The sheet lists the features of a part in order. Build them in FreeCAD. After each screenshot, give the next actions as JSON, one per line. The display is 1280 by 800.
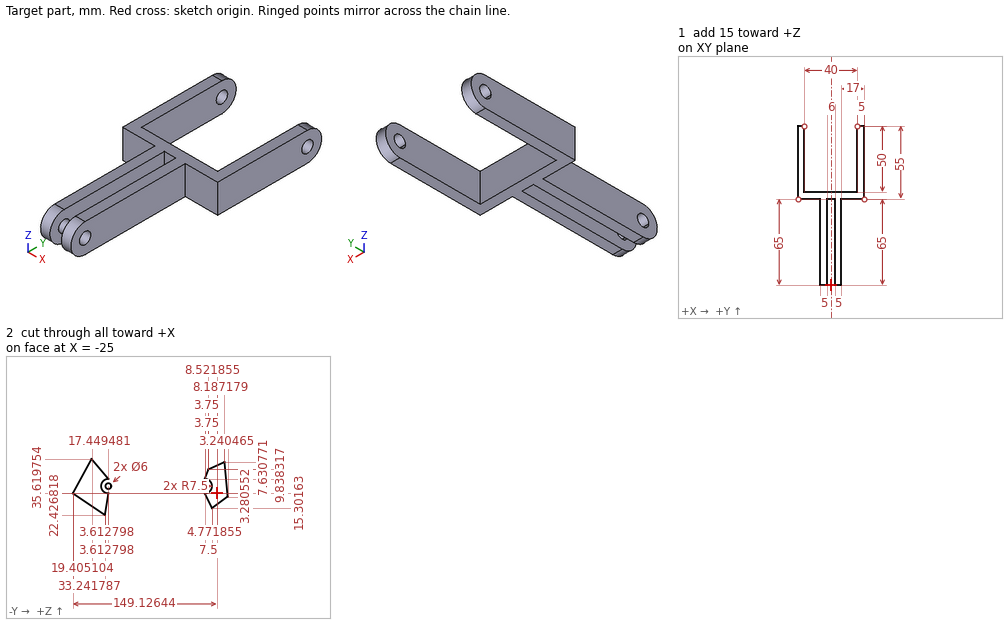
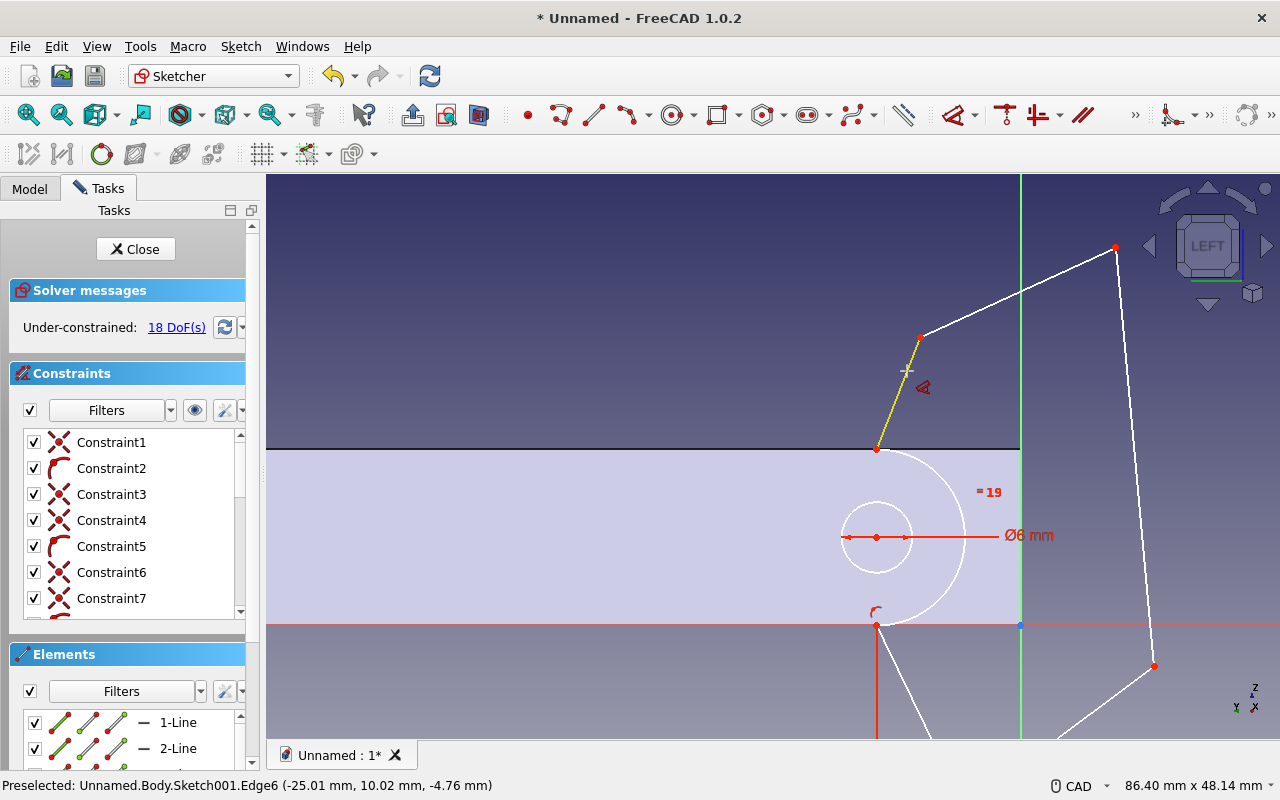
{"action": "left_click", "coordinate": [907, 371]}
{"action": "left_click", "coordinate": [898, 304]}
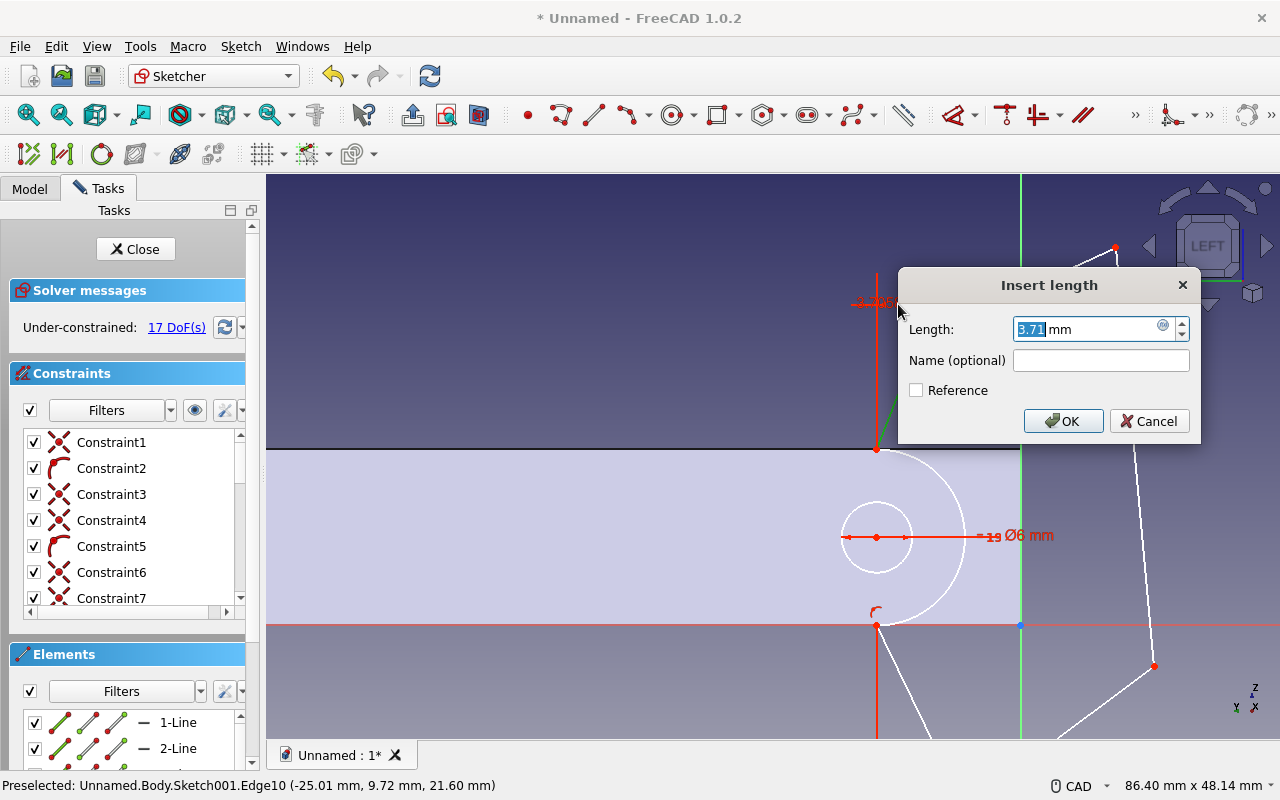
{"action": "type", "text": "3.75"}
{"action": "key", "text": "Return"}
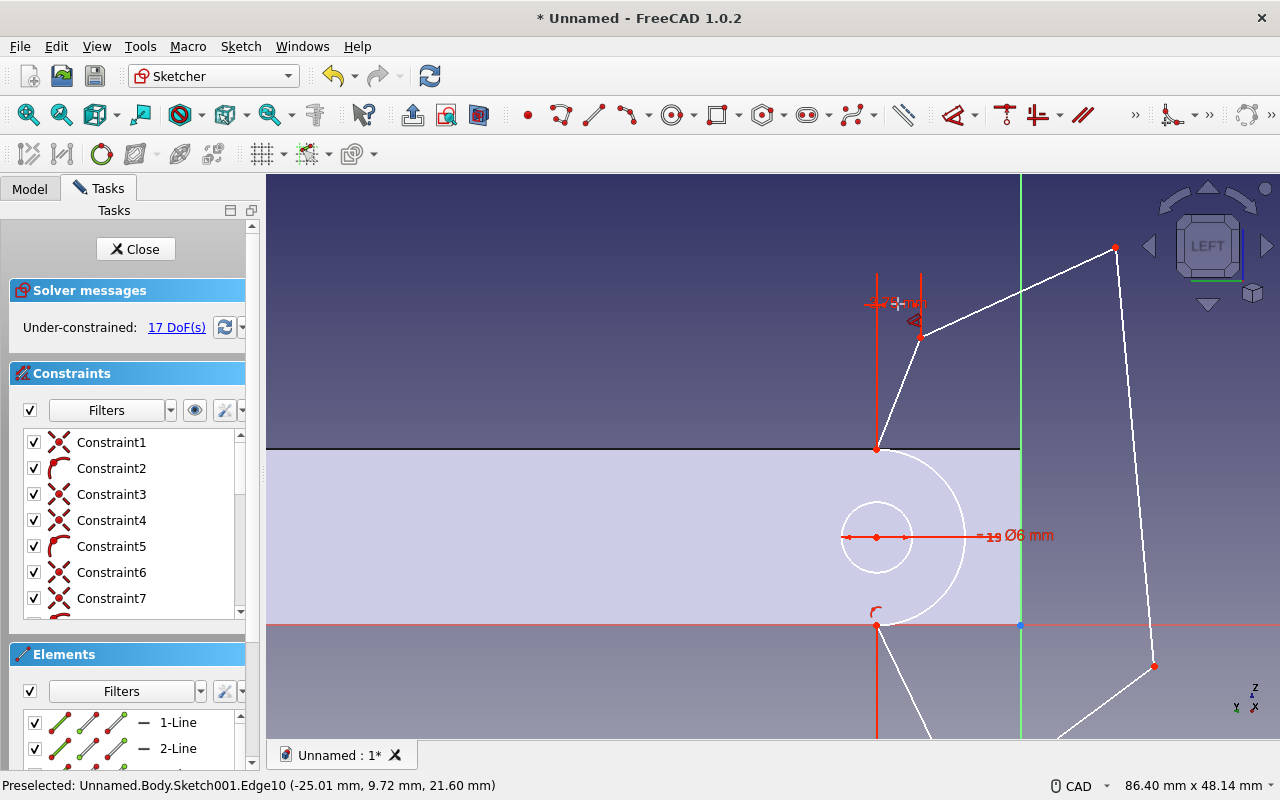
{"action": "left_click", "coordinate": [921, 338]}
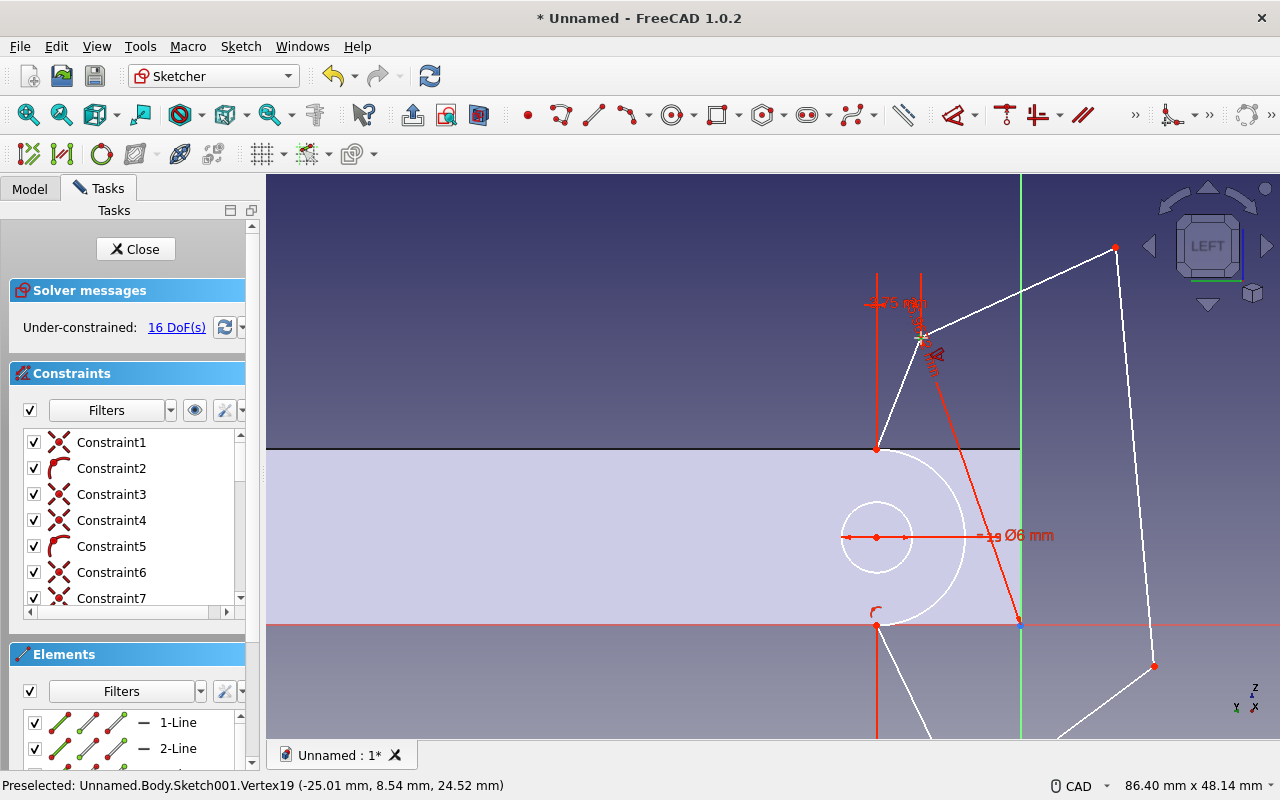
{"action": "left_click", "coordinate": [877, 537]}
{"action": "left_click", "coordinate": [914, 571]}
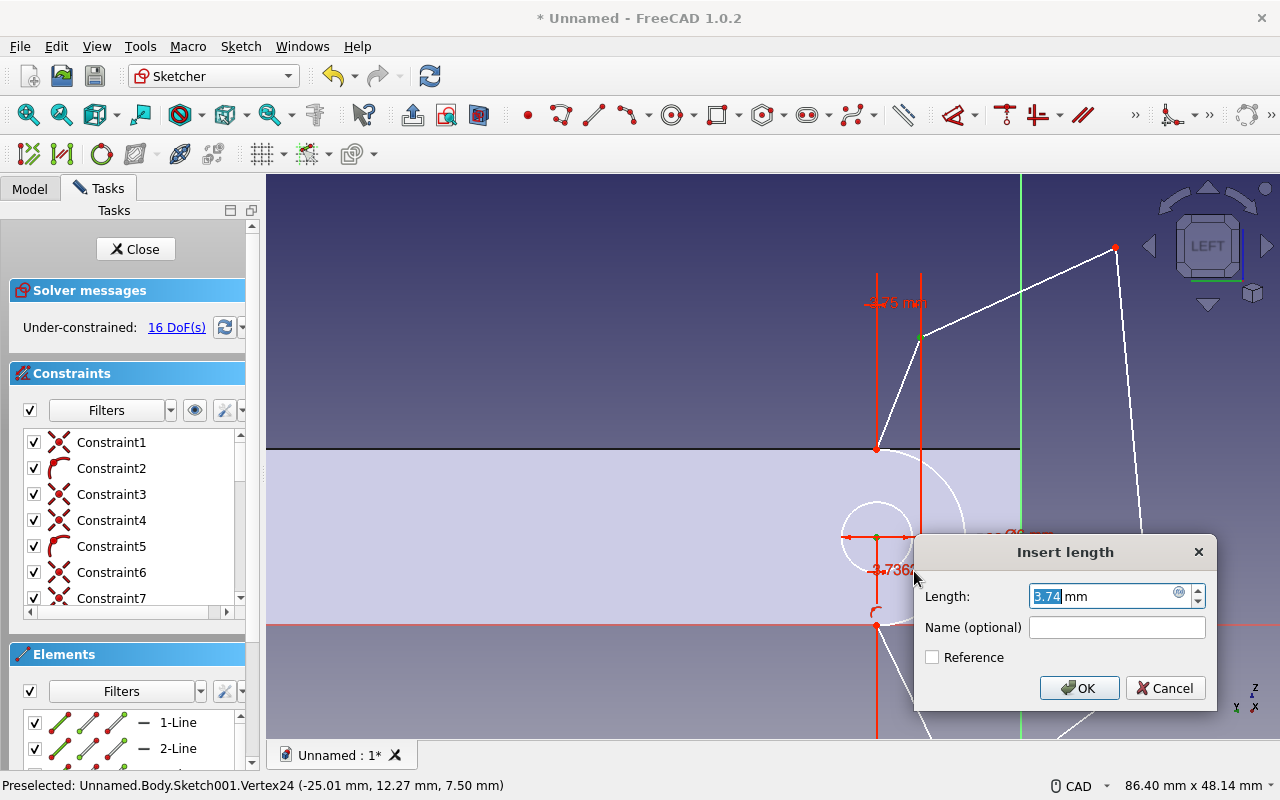
{"action": "type", "text": "3.75"}
{"action": "key", "text": "Return"}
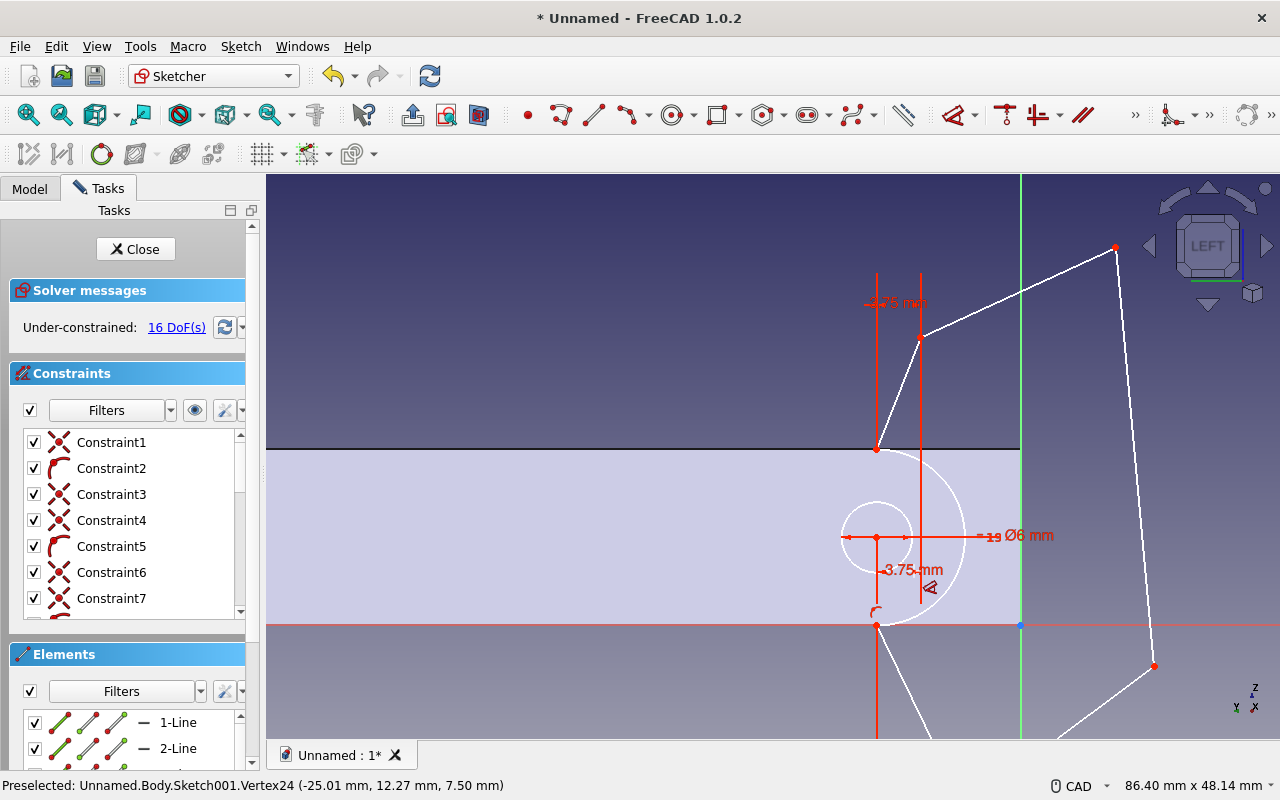
{"action": "scroll", "coordinate": [916, 417], "scroll_direction": "down", "scroll_amount": 6}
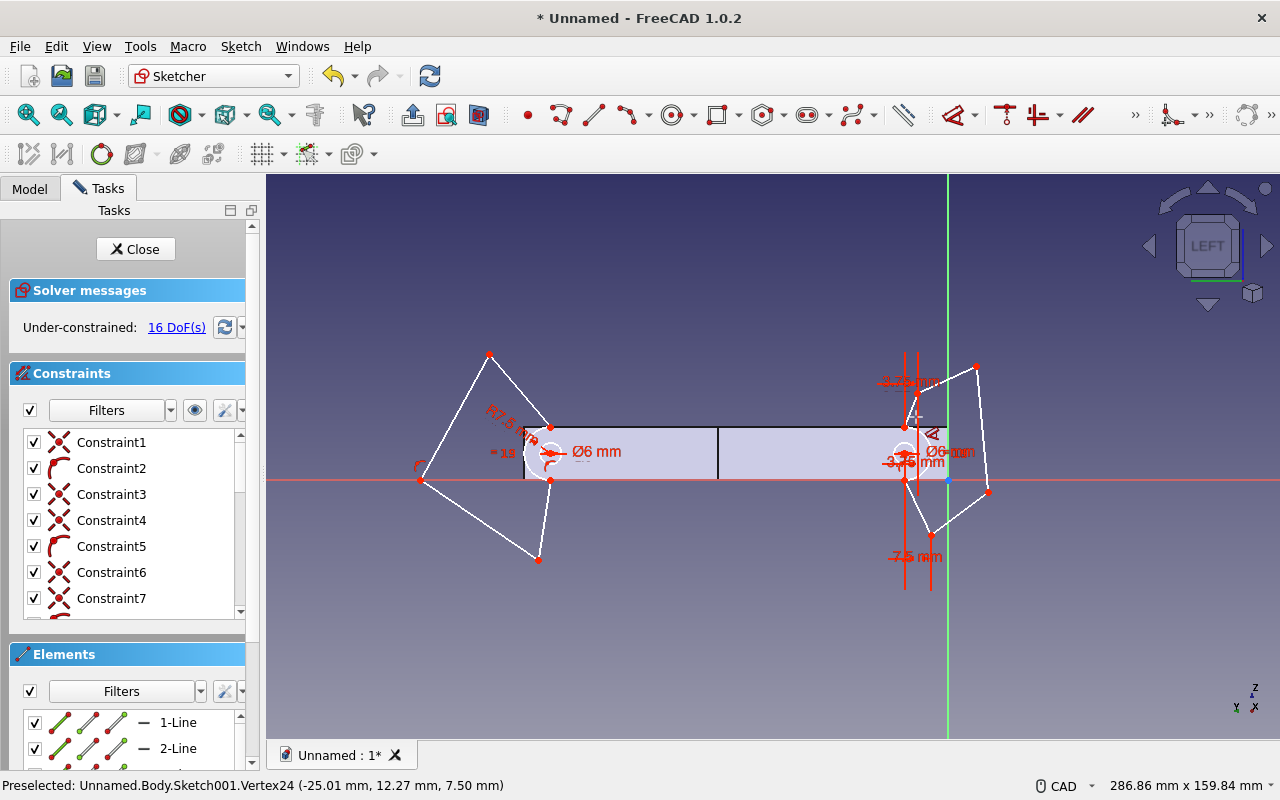
{"action": "scroll", "coordinate": [931, 535], "scroll_direction": "up", "scroll_amount": 5}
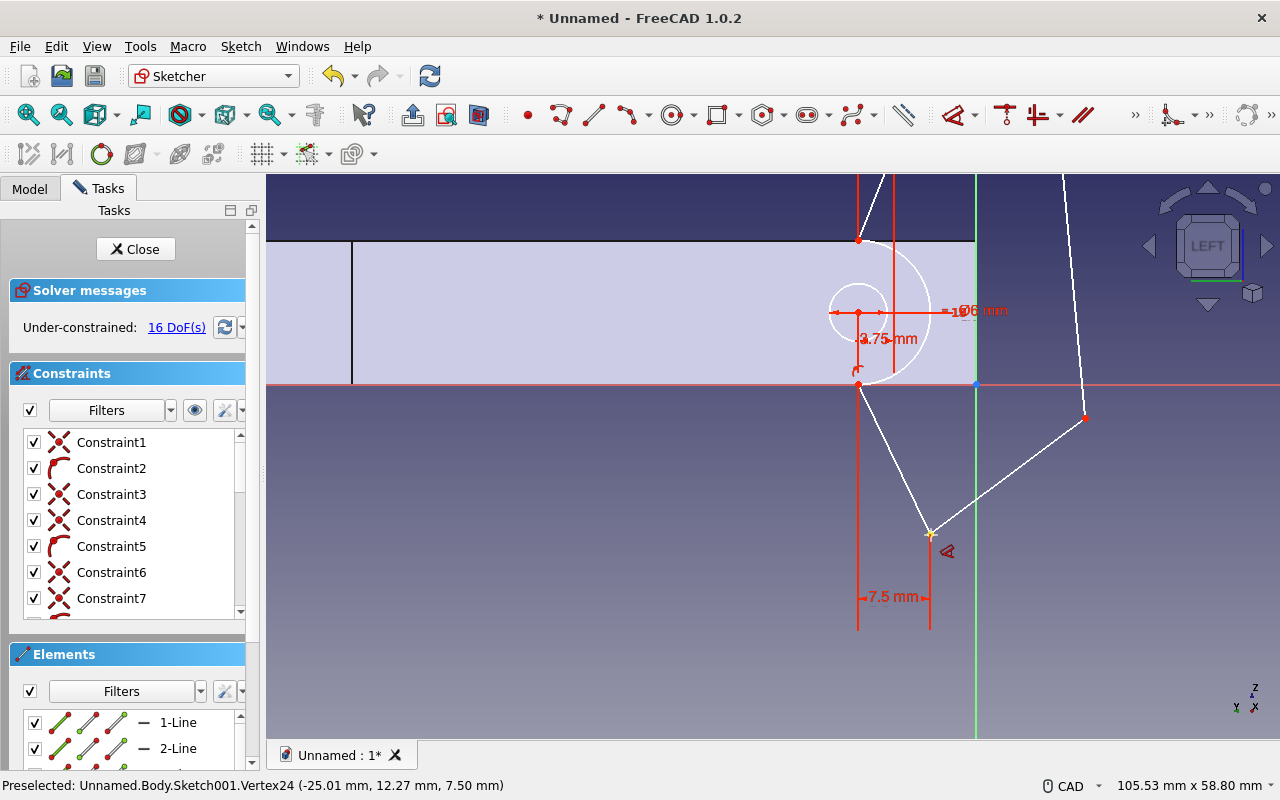
{"action": "left_click", "coordinate": [930, 534]}
{"action": "left_click", "coordinate": [953, 568]}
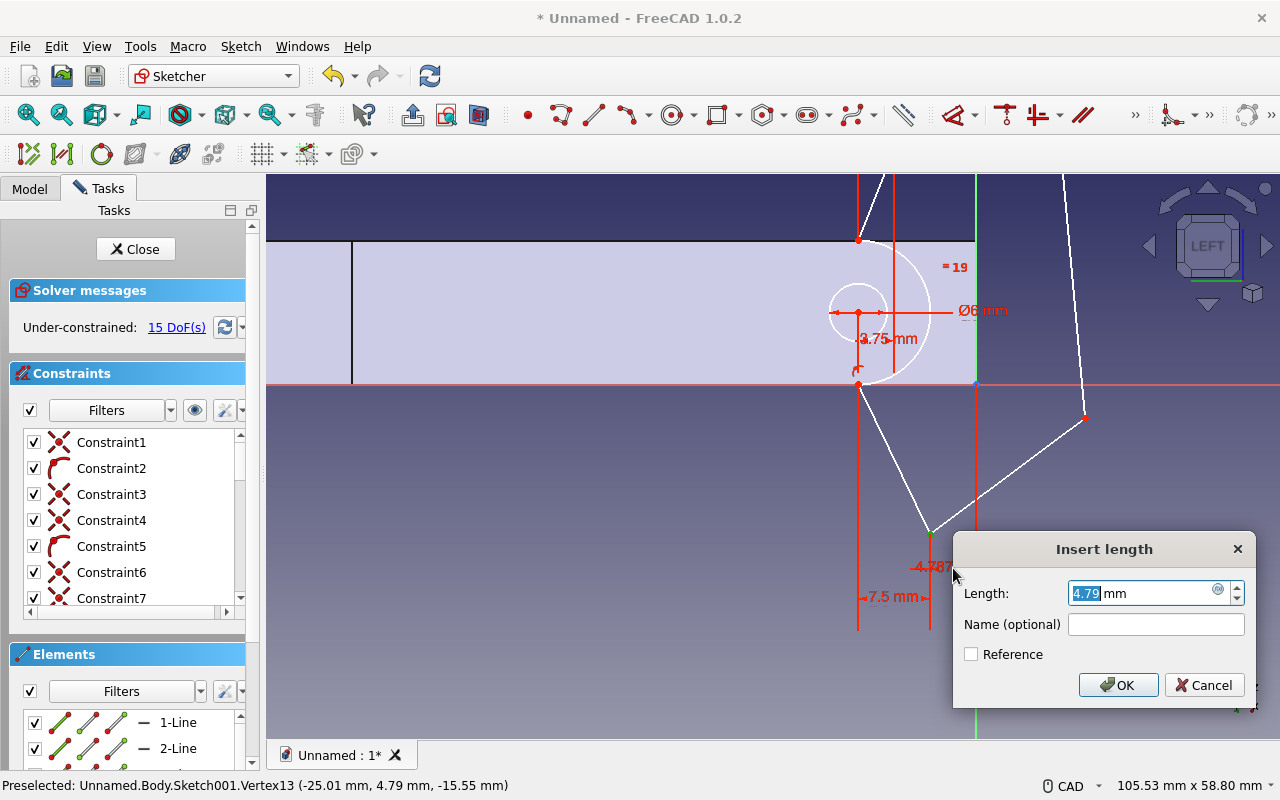
{"action": "type", "text": "4.771855"}
{"action": "key", "text": "Return"}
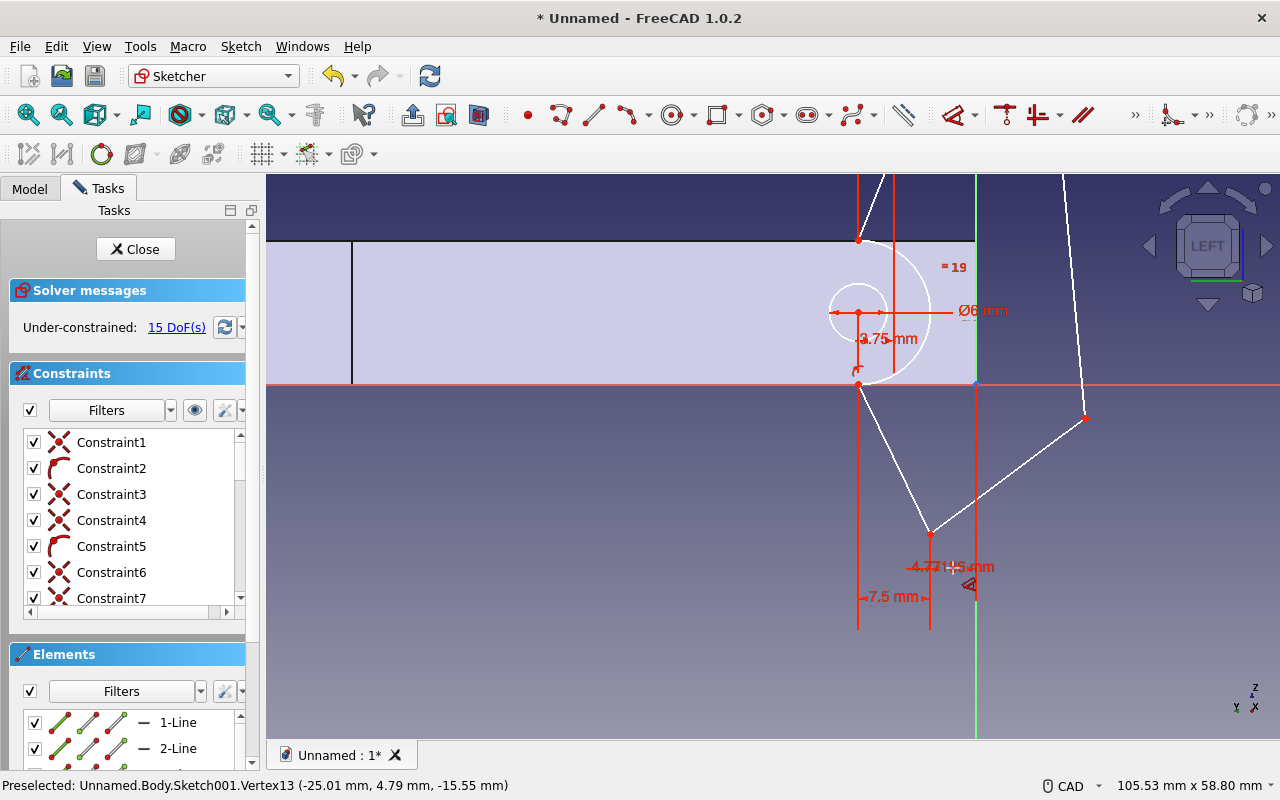
{"action": "left_click", "coordinate": [930, 534]}
{"action": "left_click", "coordinate": [1010, 425]}